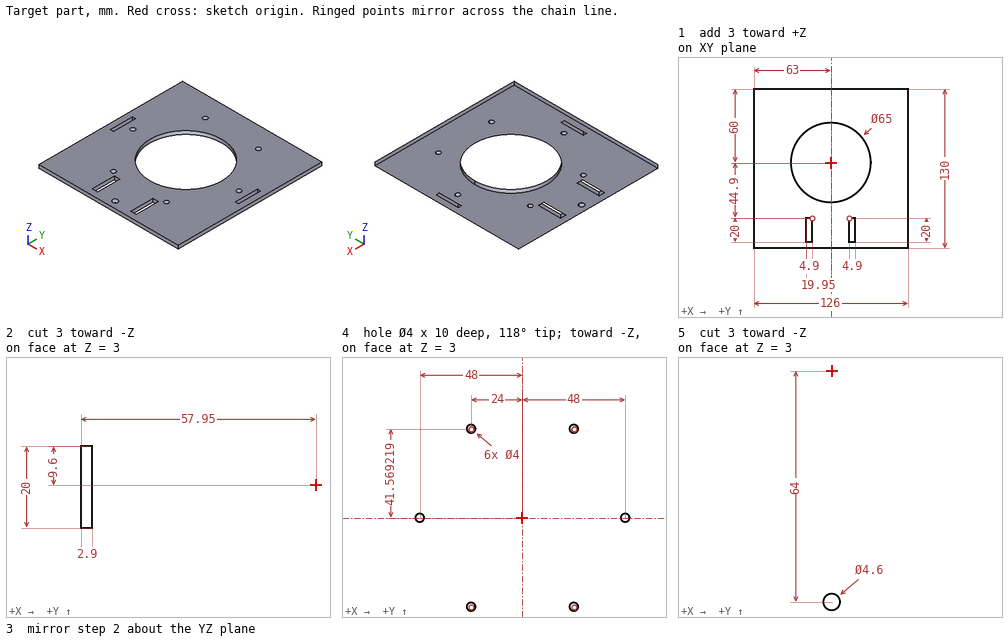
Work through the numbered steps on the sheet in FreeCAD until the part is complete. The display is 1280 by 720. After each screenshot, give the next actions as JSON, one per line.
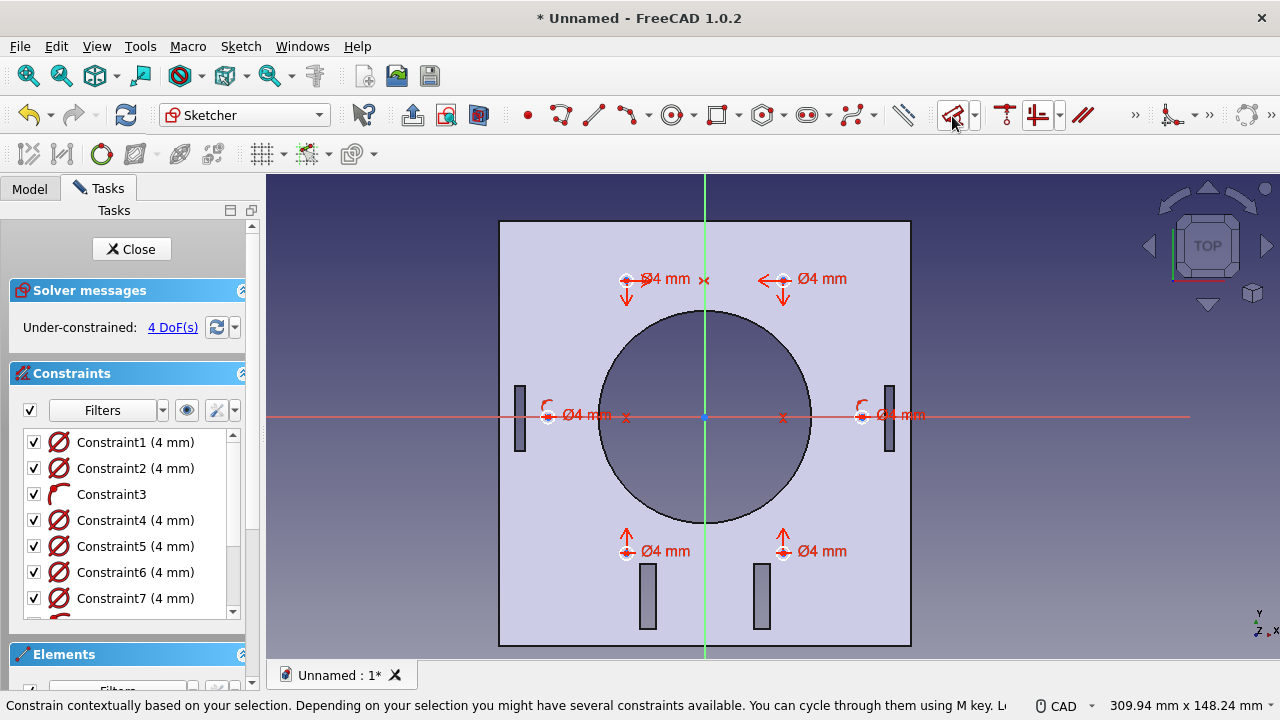
{"action": "left_click", "coordinate": [627, 281]}
{"action": "left_click", "coordinate": [666, 247]}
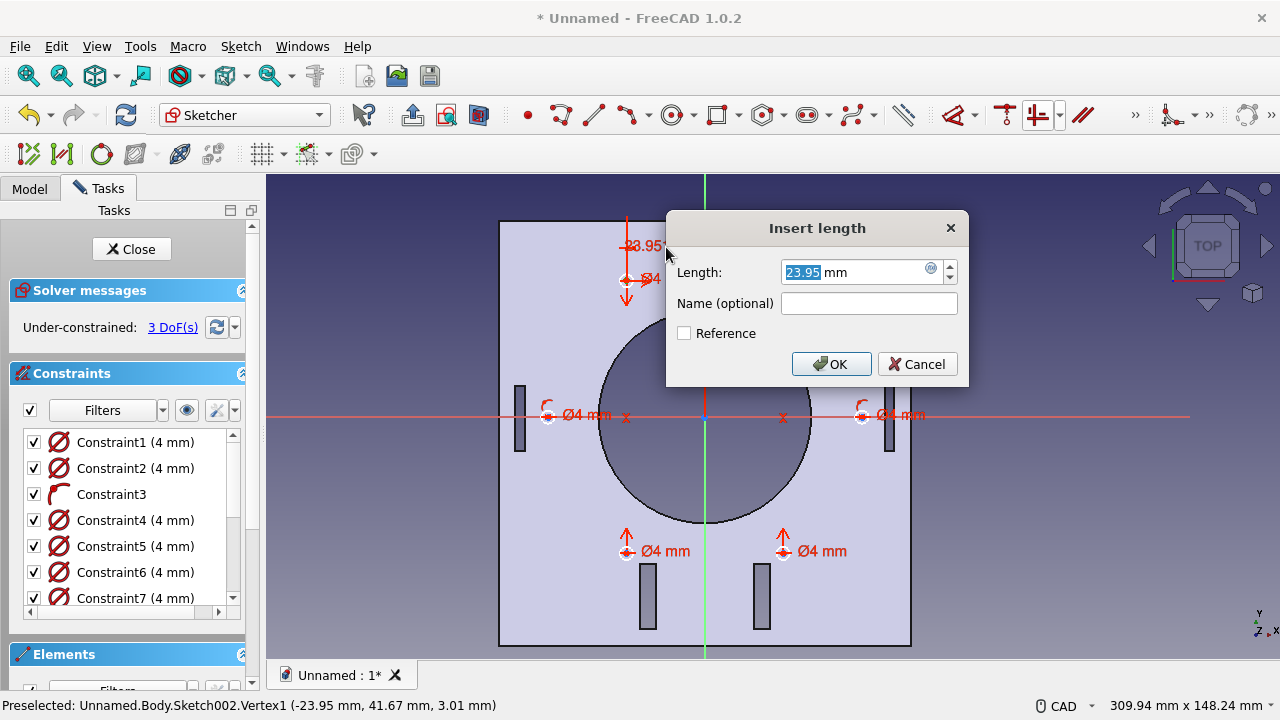
{"action": "type", "text": "24"}
{"action": "key", "text": "Return"}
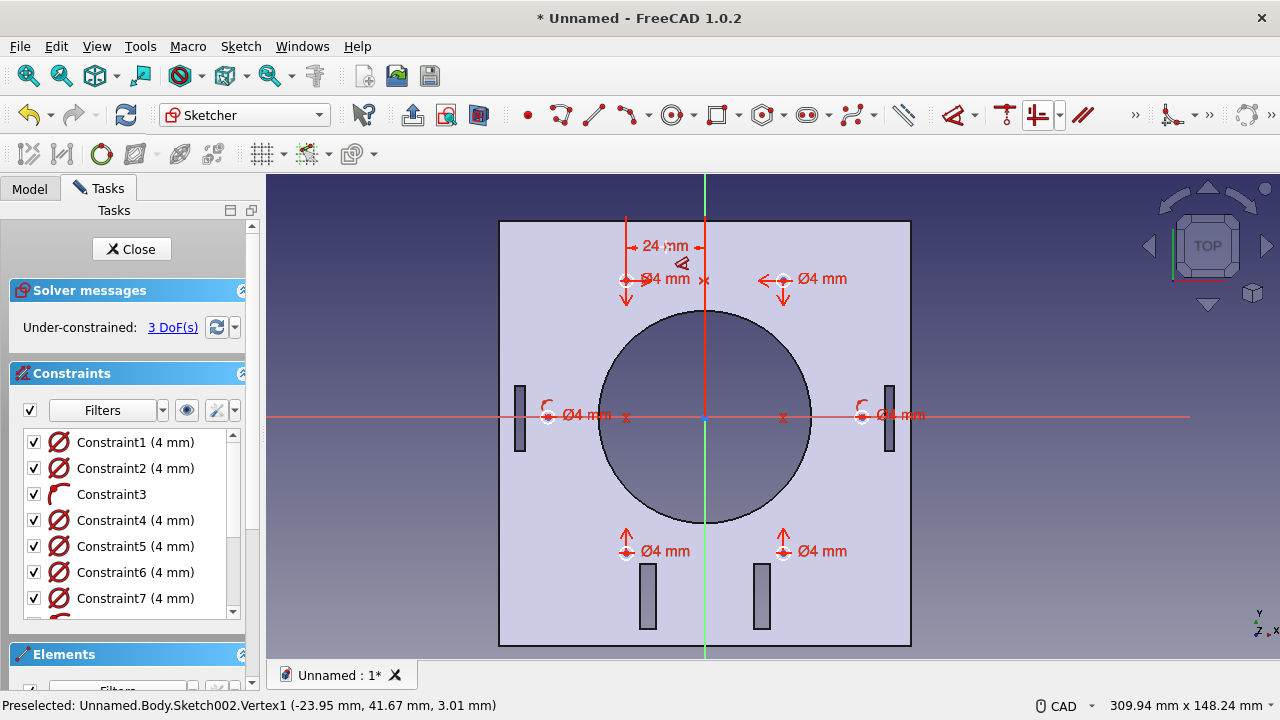
{"action": "left_click", "coordinate": [862, 417]}
{"action": "left_click", "coordinate": [783, 451]}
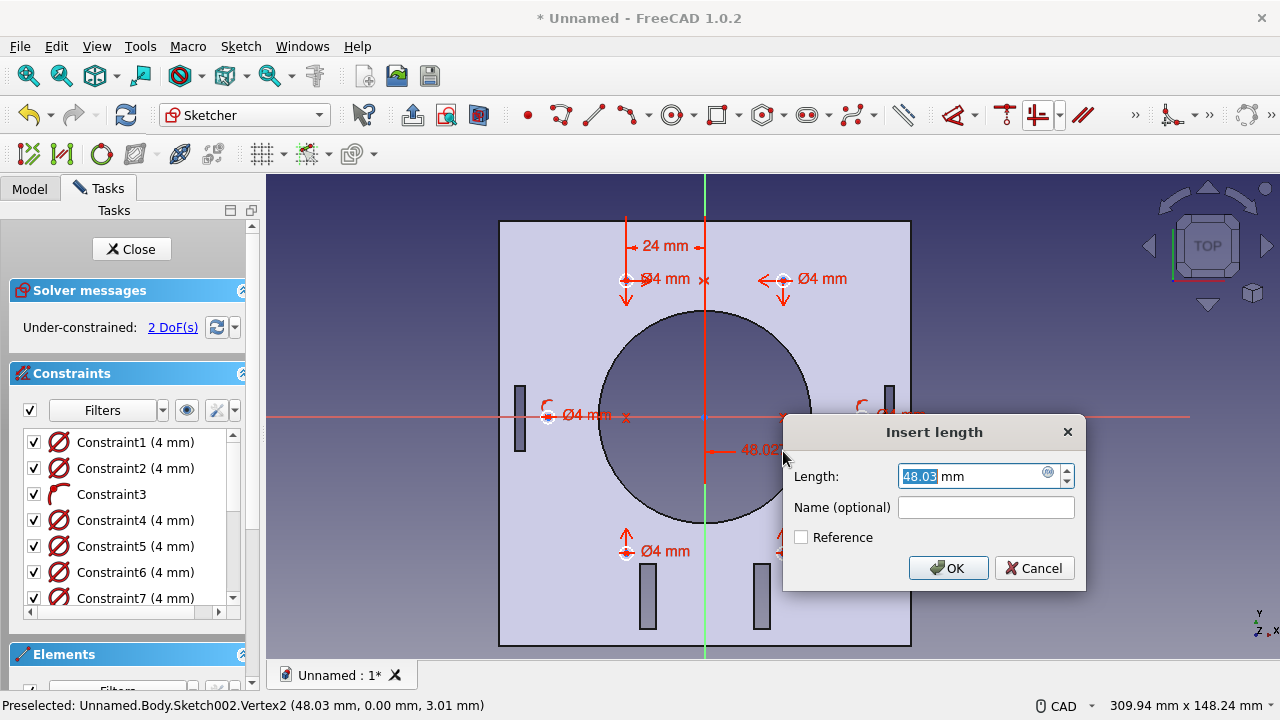
{"action": "type", "text": "48"}
{"action": "key", "text": "Return"}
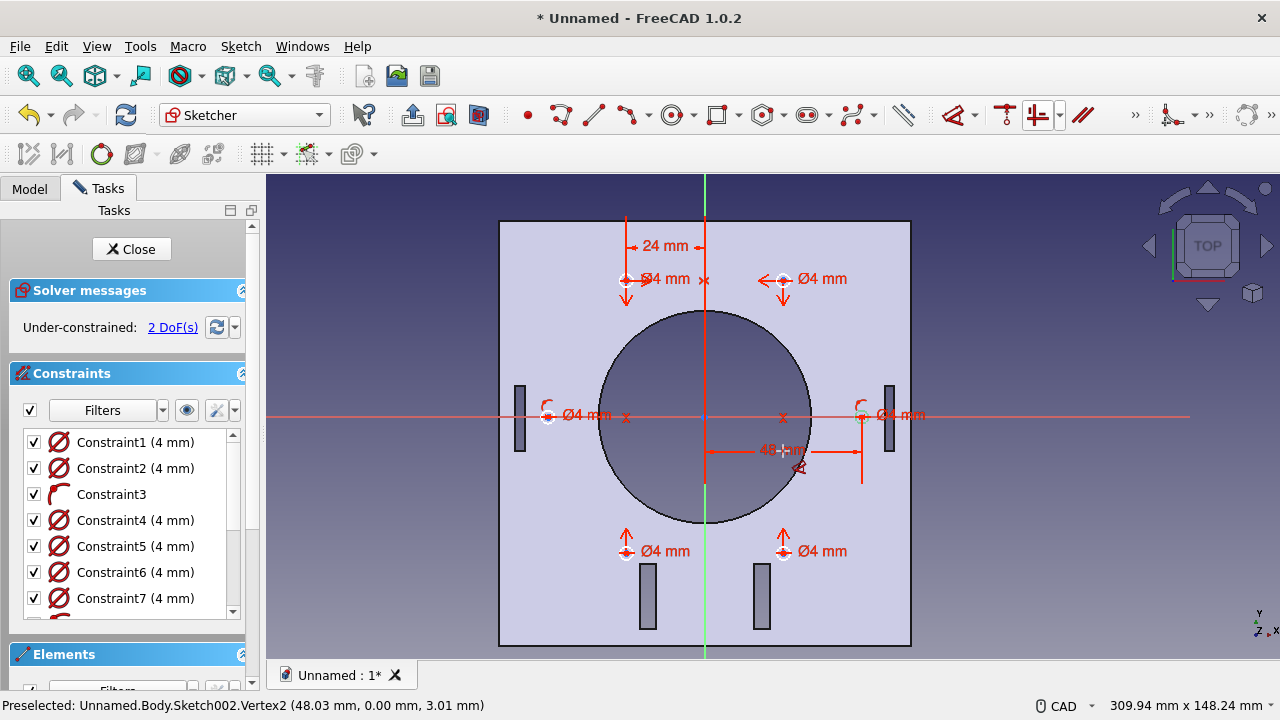
{"action": "left_click", "coordinate": [548, 417]}
{"action": "left_click", "coordinate": [626, 451]}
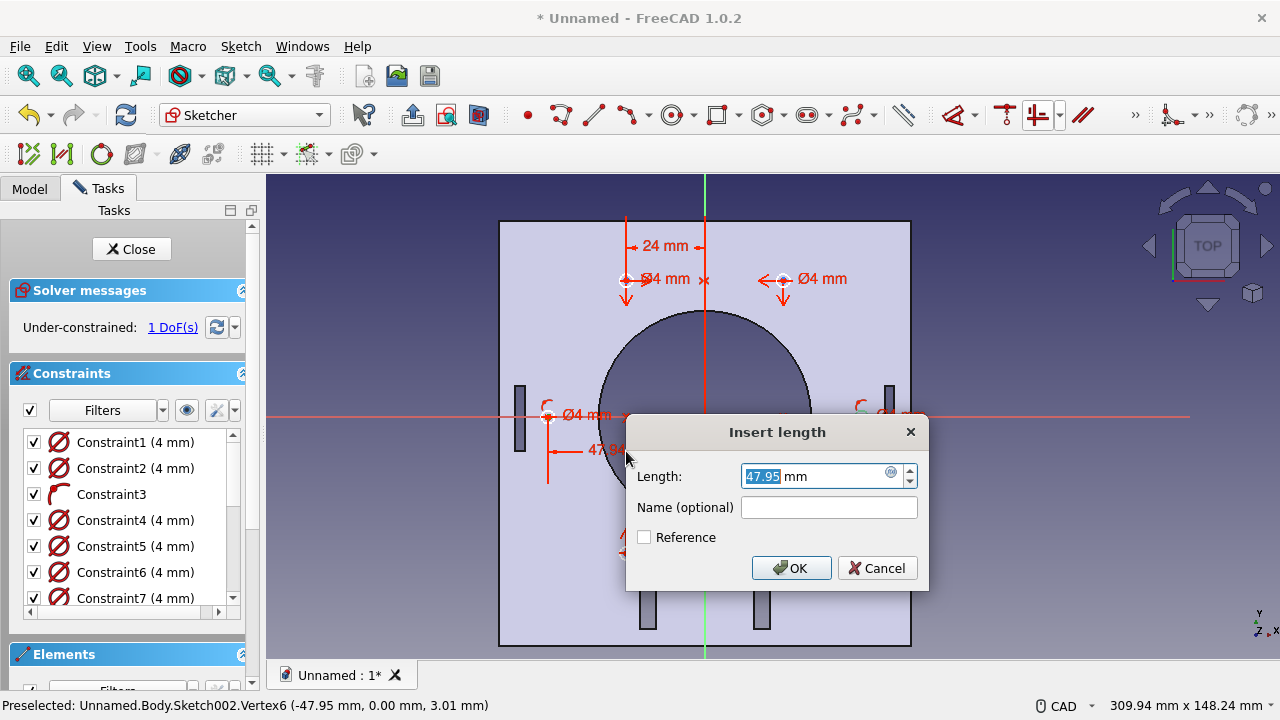
{"action": "type", "text": "48"}
{"action": "key", "text": "Return"}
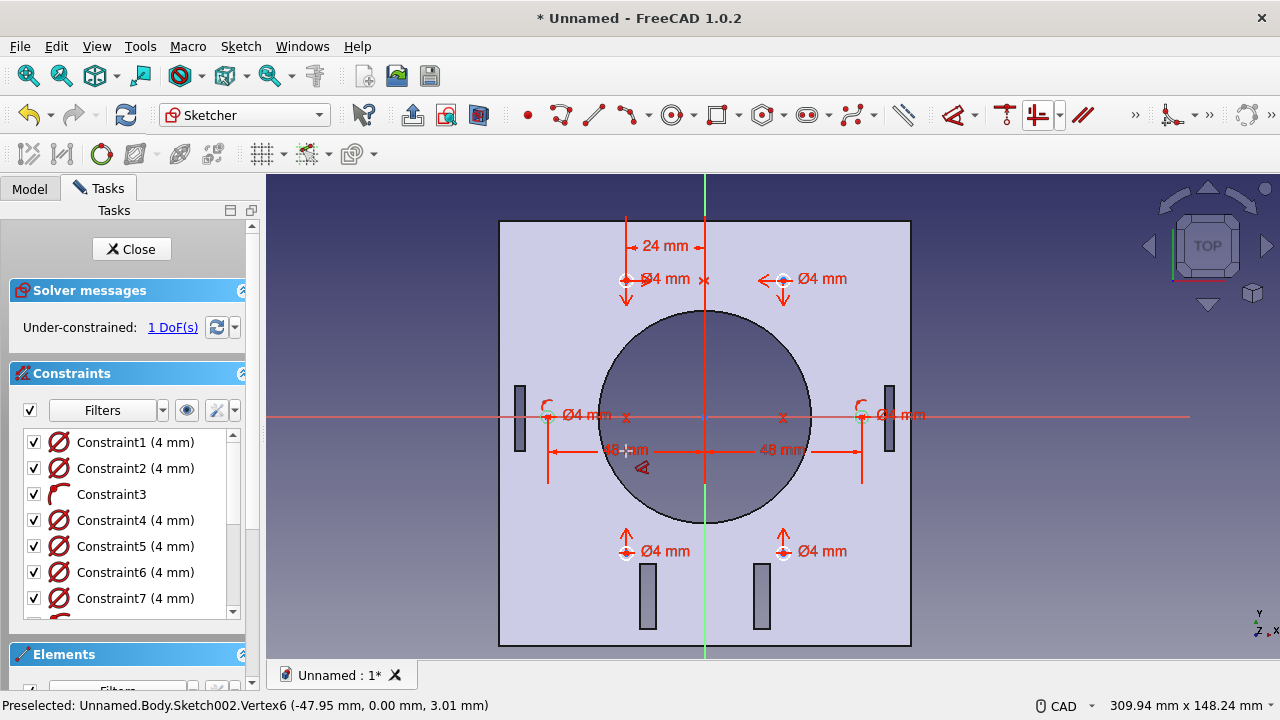
{"action": "left_click", "coordinate": [626, 281]}
{"action": "left_click", "coordinate": [592, 349]}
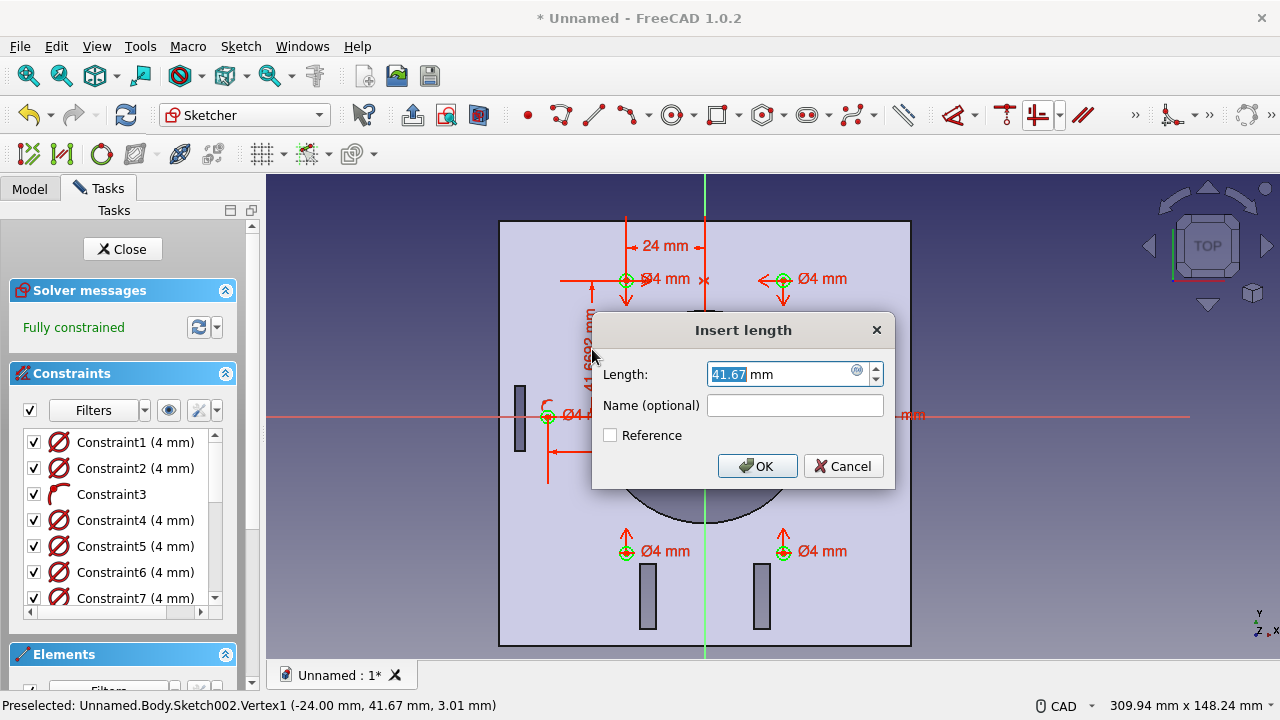
{"action": "type", "text": "41.569219"}
{"action": "key", "text": "Return"}
{"action": "key", "text": "Escape"}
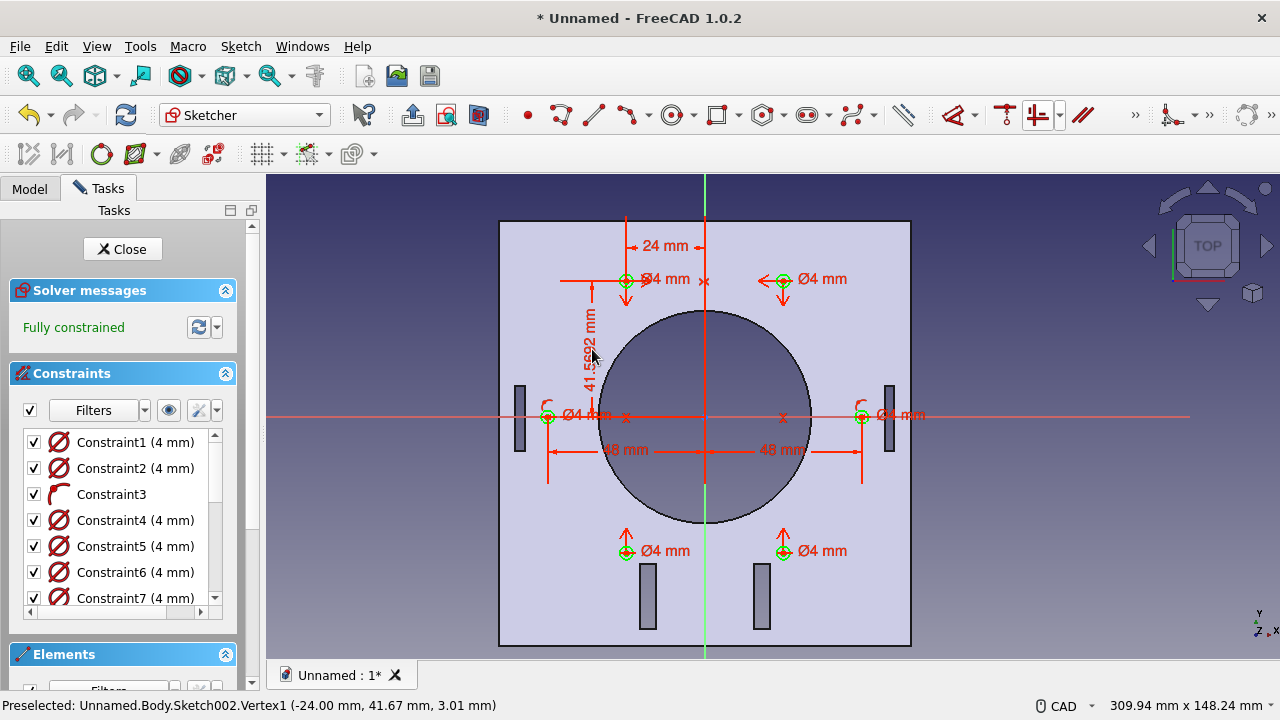
{"action": "left_click", "coordinate": [123, 249]}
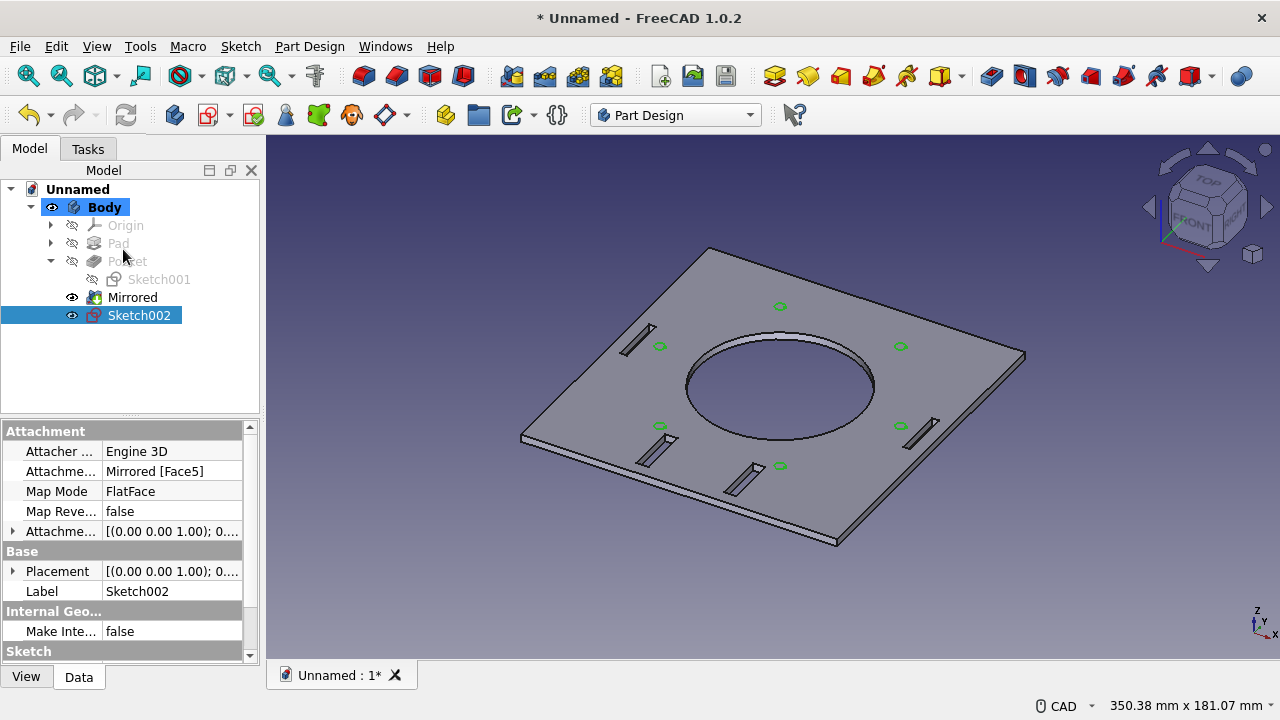
{"action": "left_click", "coordinate": [1025, 76]}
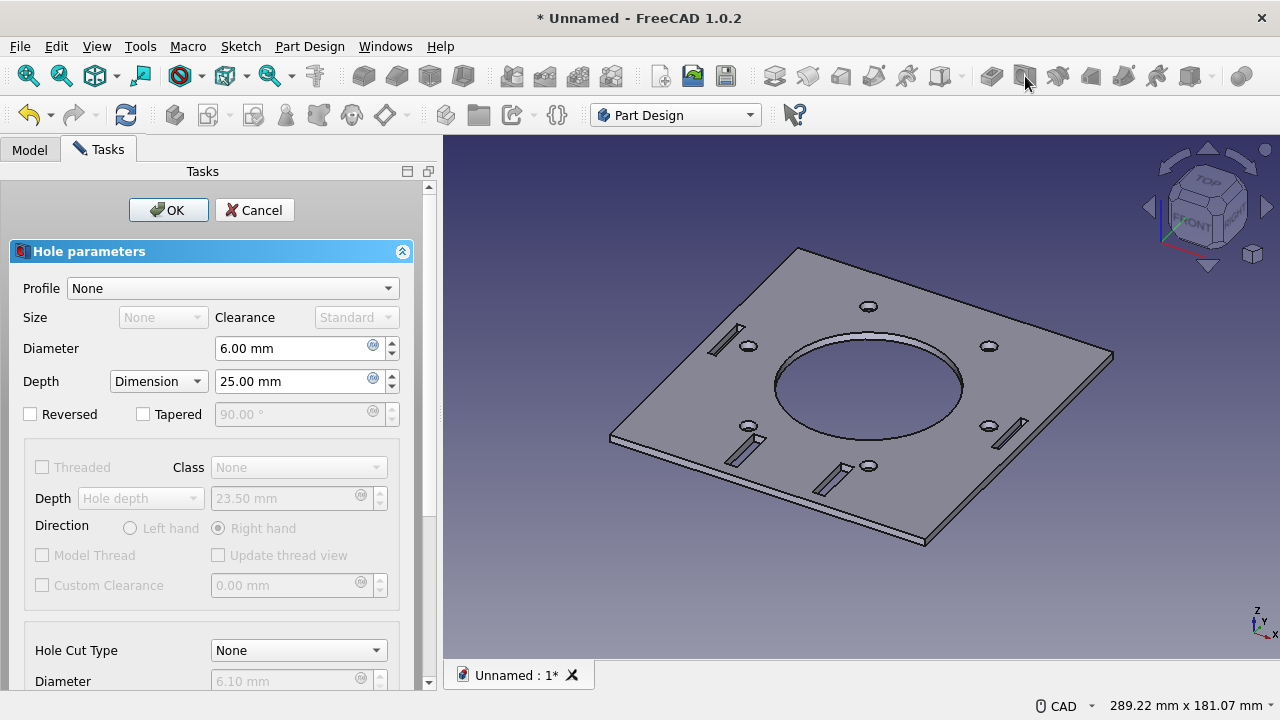
{"action": "triple_click", "coordinate": [300, 348]}